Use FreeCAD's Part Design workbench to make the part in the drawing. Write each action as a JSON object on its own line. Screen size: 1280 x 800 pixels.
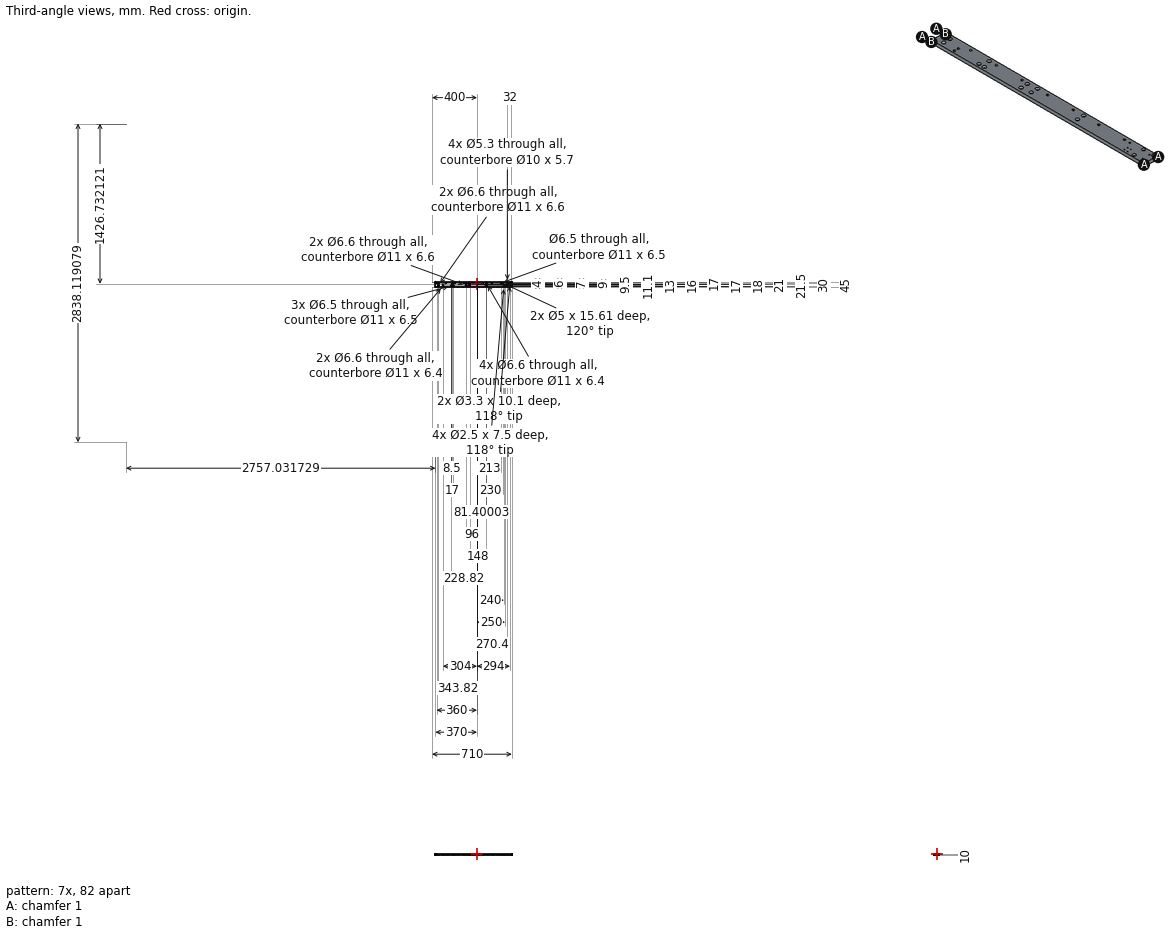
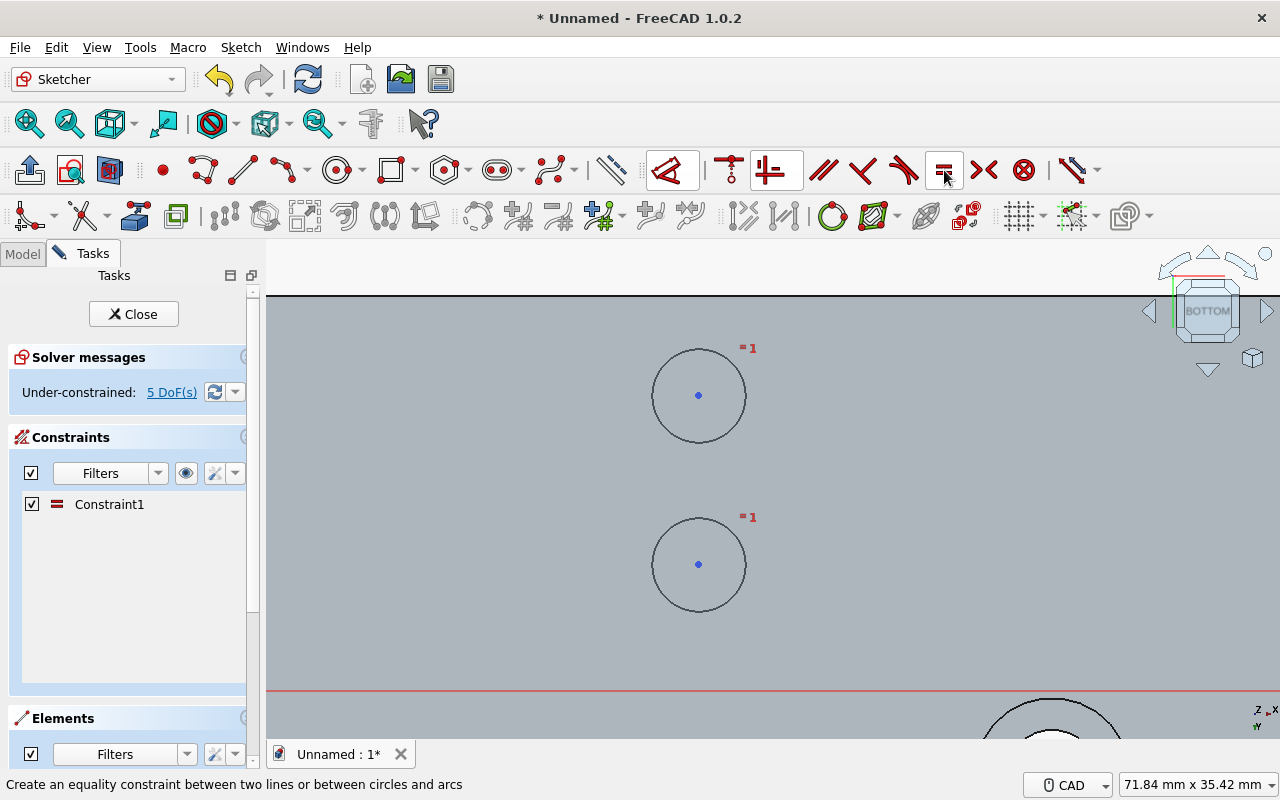
{"action": "left_click", "coordinate": [699, 396]}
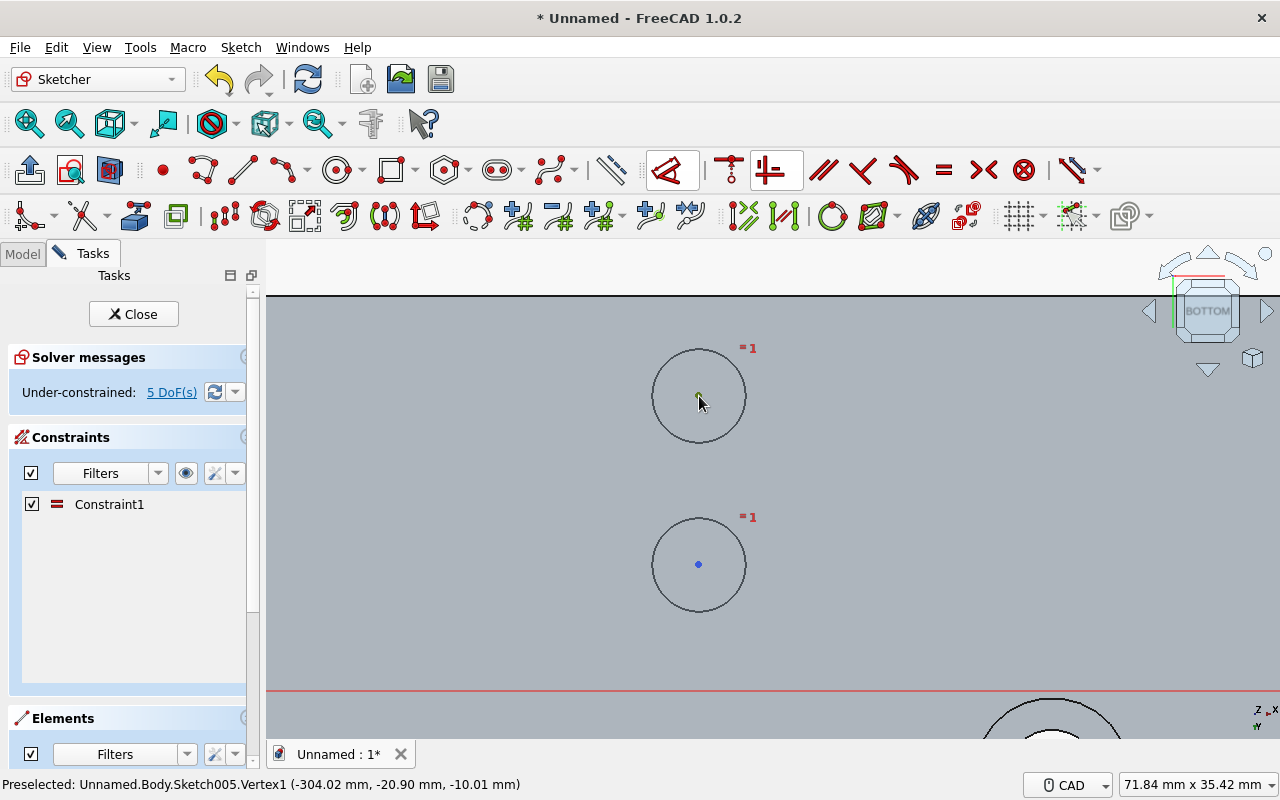
{"action": "left_click", "coordinate": [699, 565]}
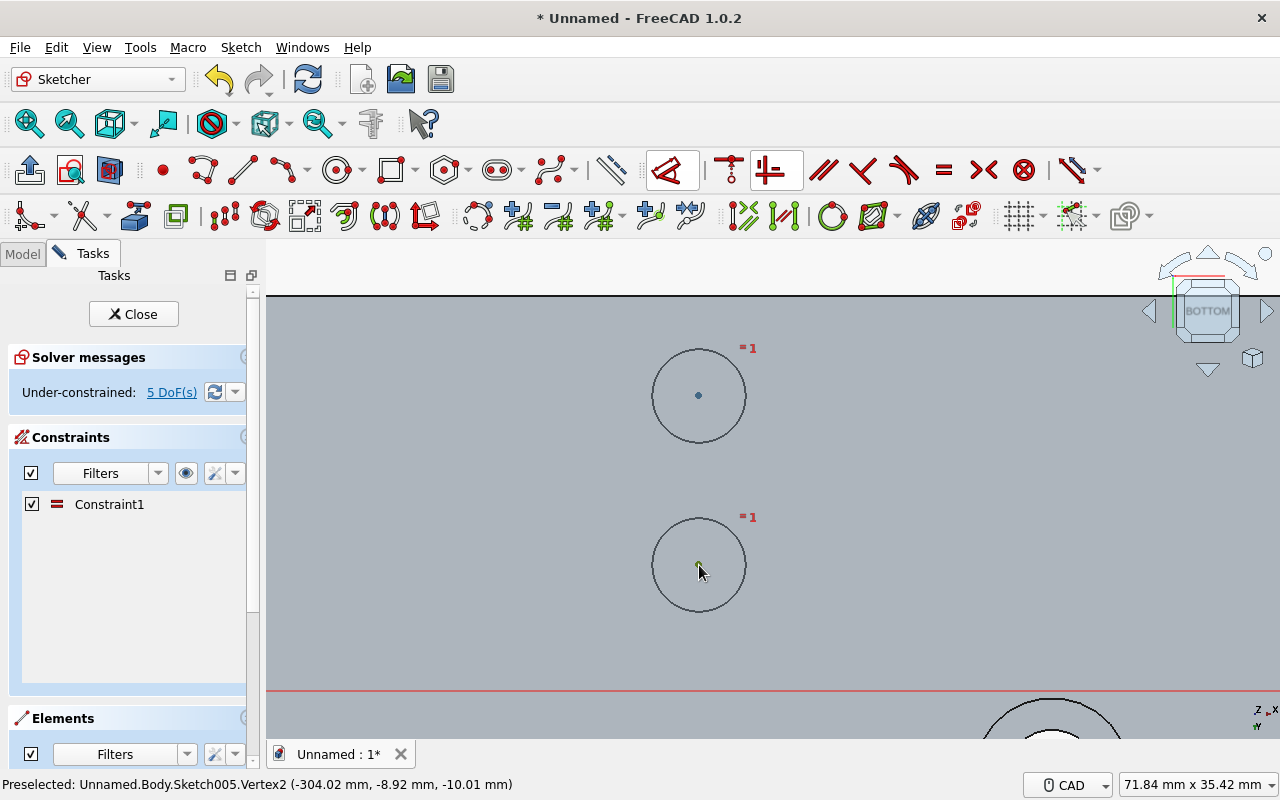
{"action": "left_click", "coordinate": [798, 170]}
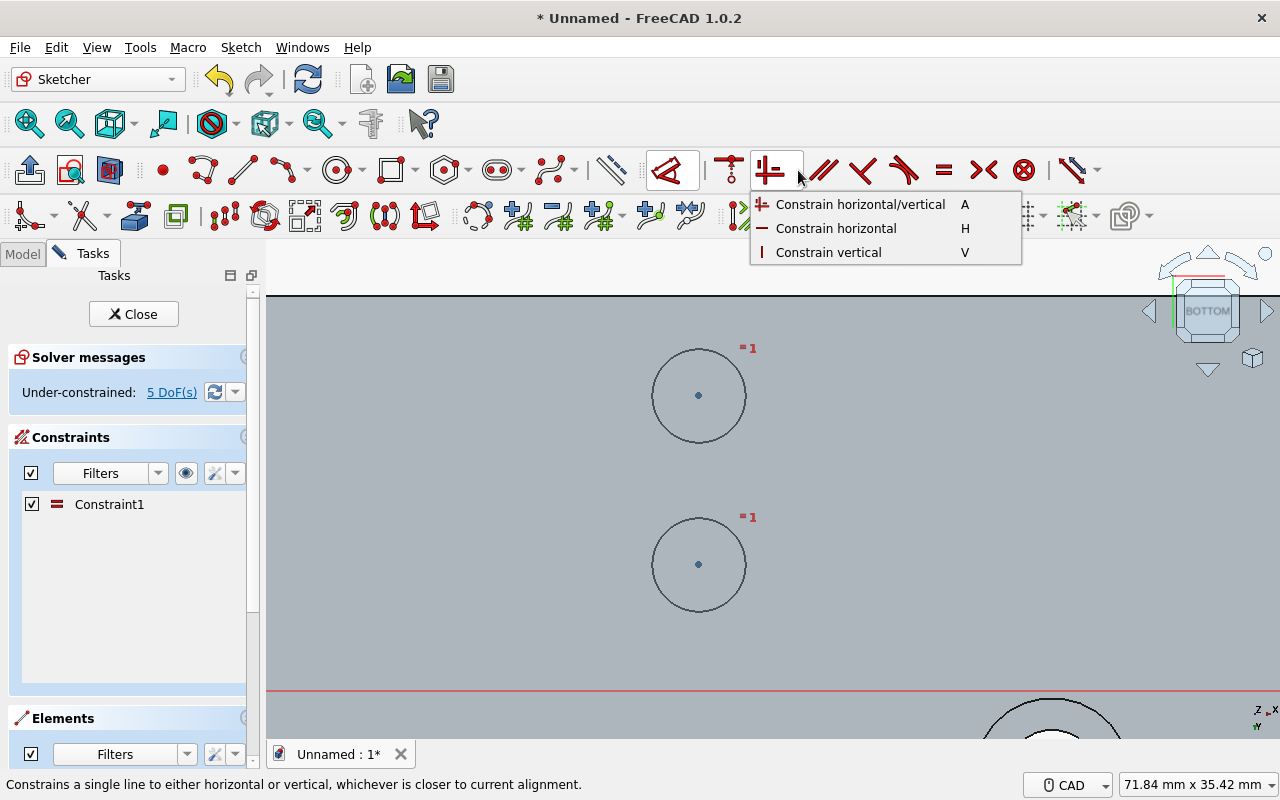
{"action": "left_click", "coordinate": [886, 252]}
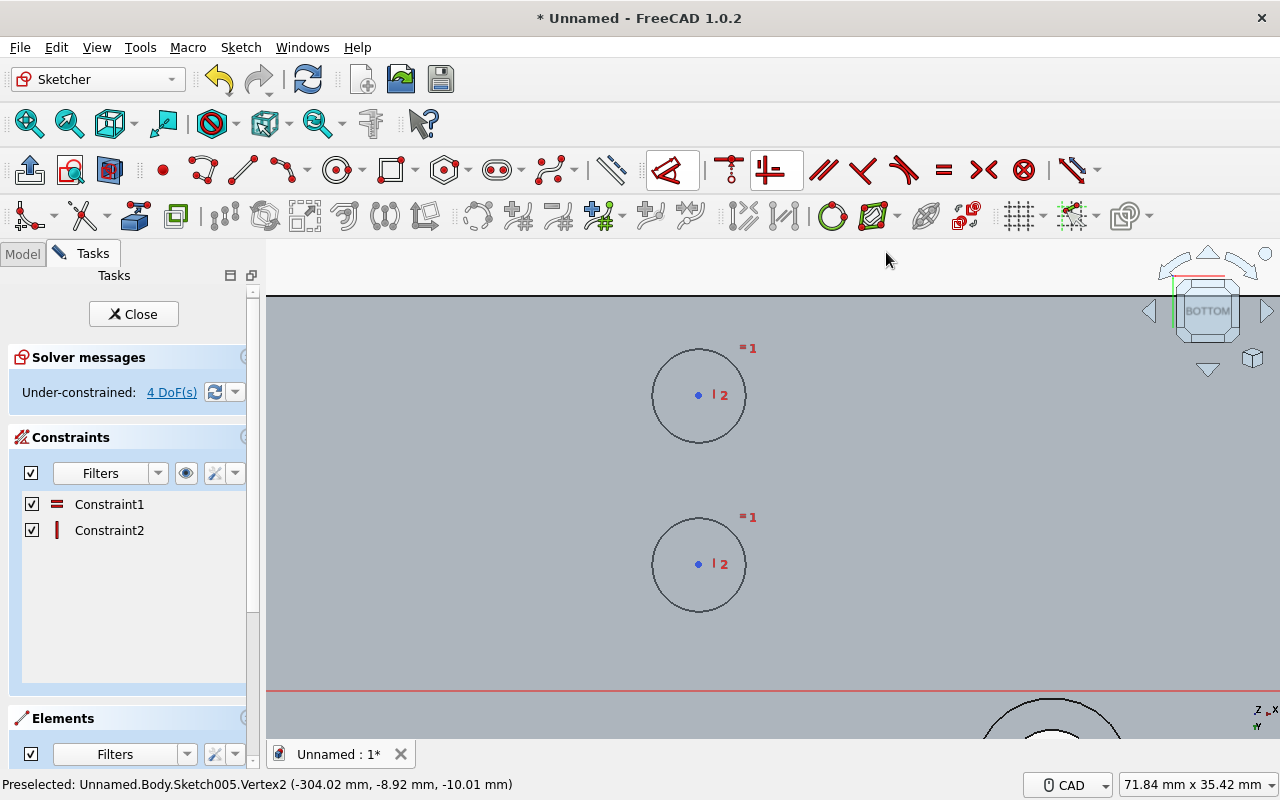
{"action": "left_click", "coordinate": [732, 363]}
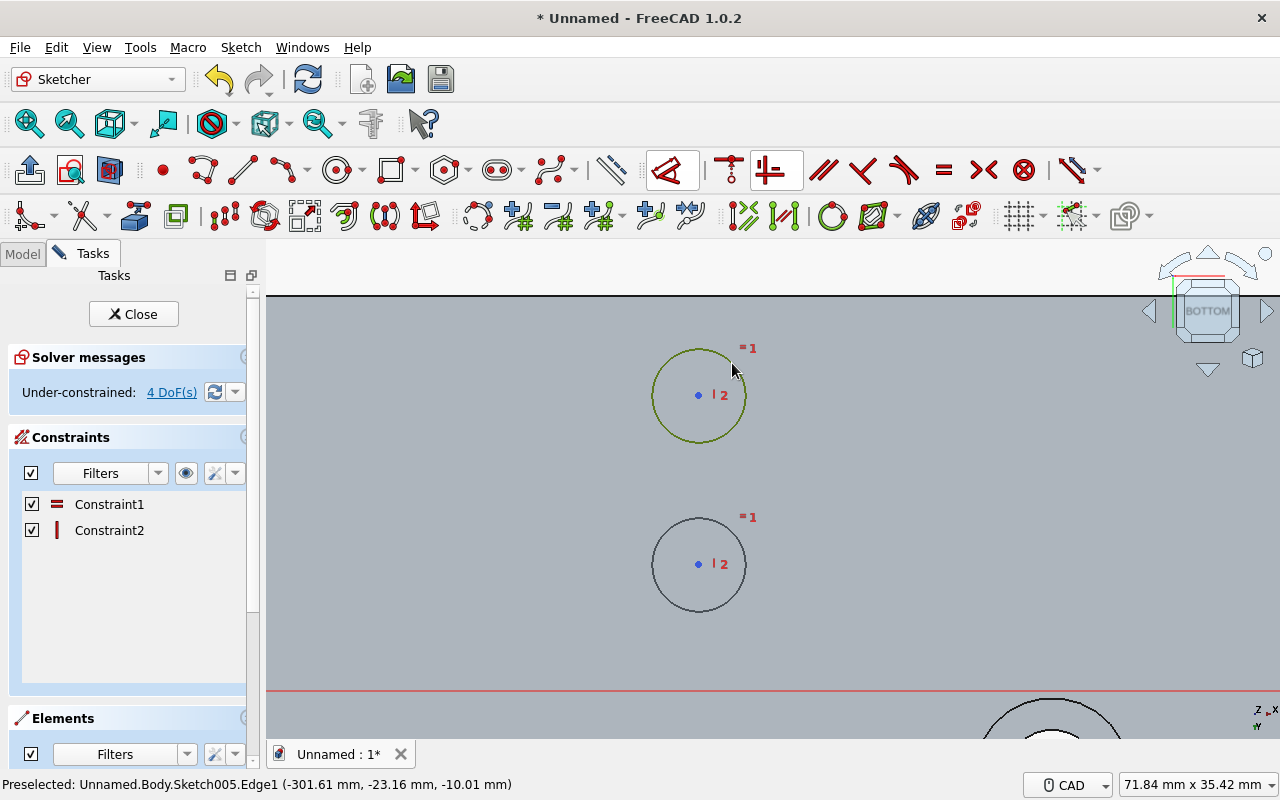
{"action": "left_click", "coordinate": [694, 170]}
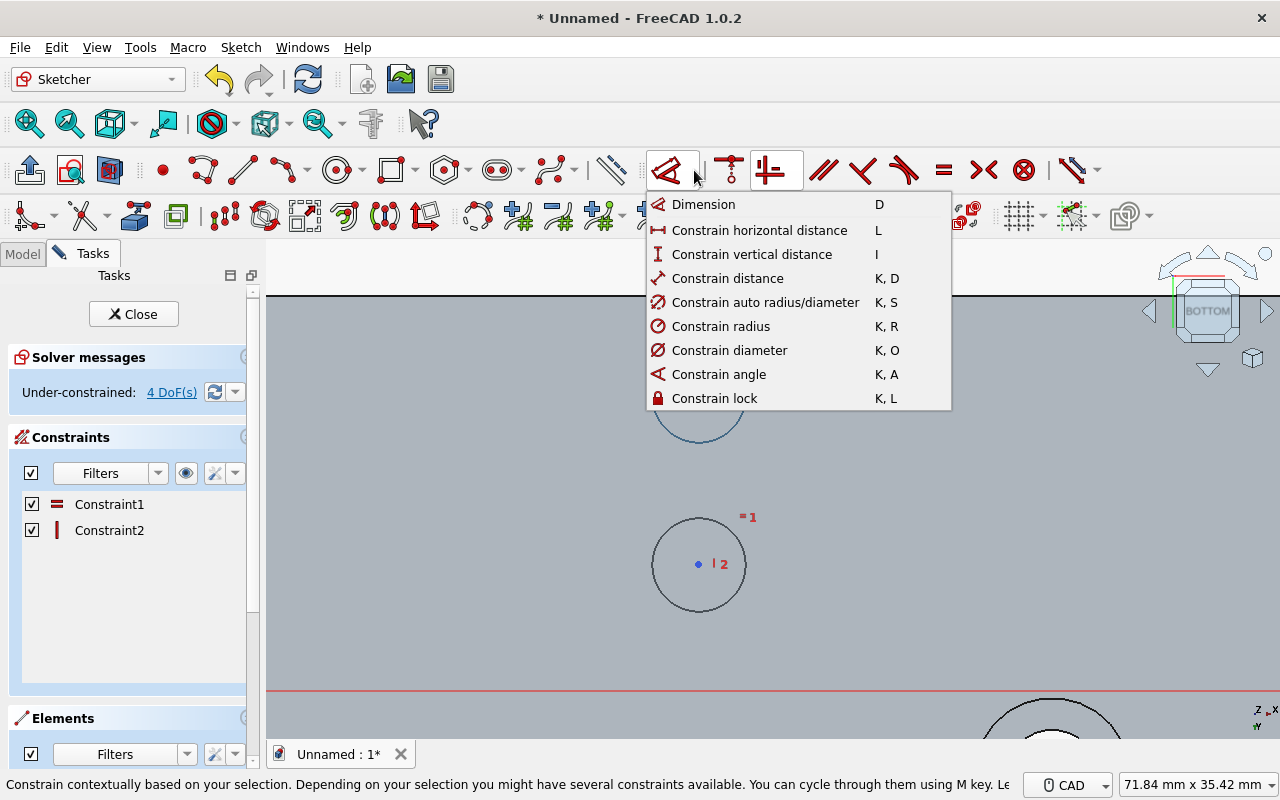
{"action": "left_click", "coordinate": [799, 350]}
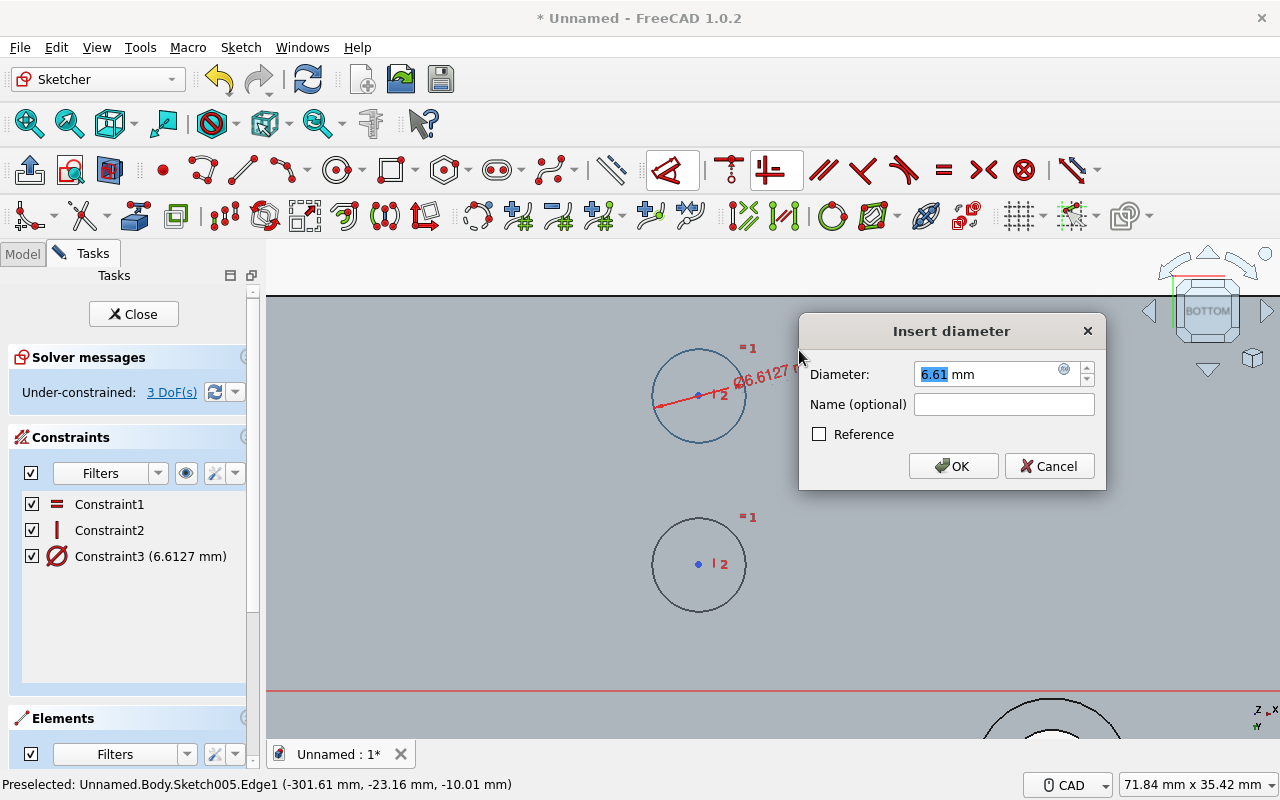
{"action": "type", "text": "6.6"}
{"action": "key", "text": "Return"}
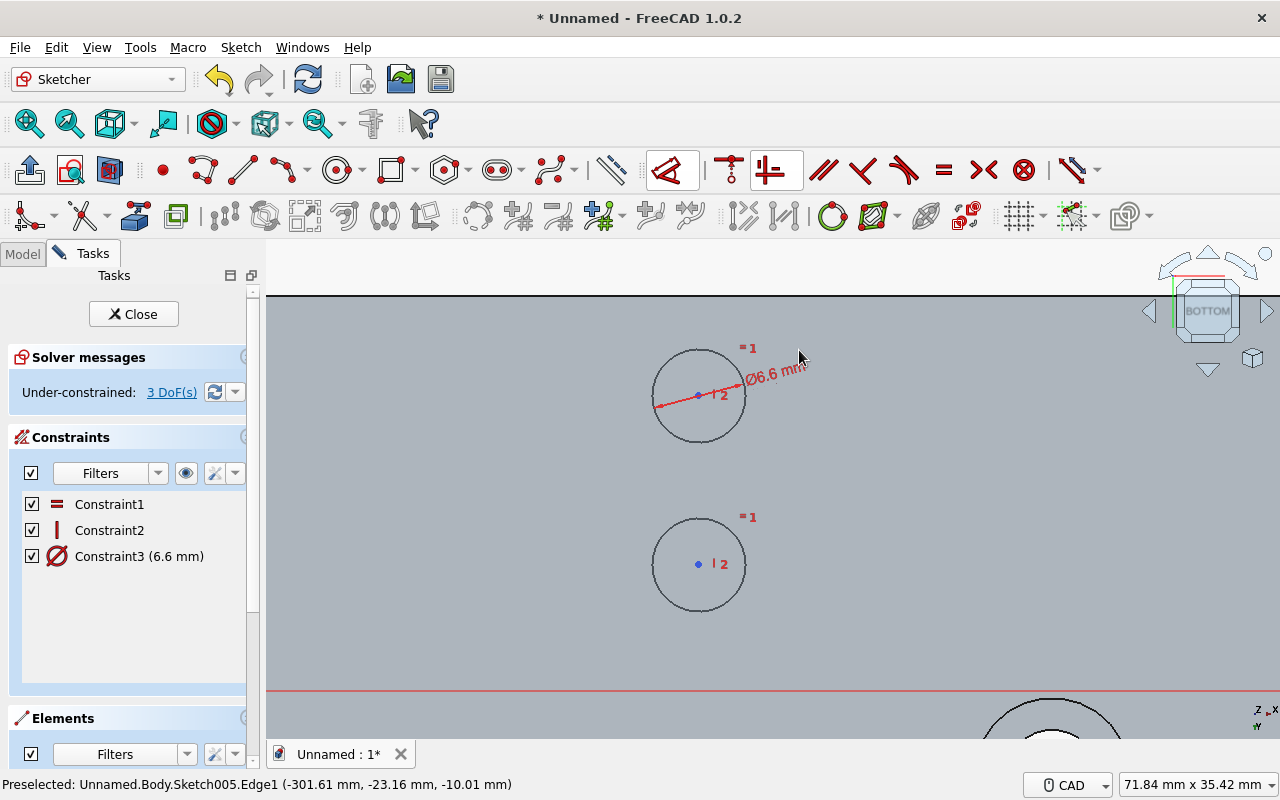
{"action": "left_click", "coordinate": [699, 565]}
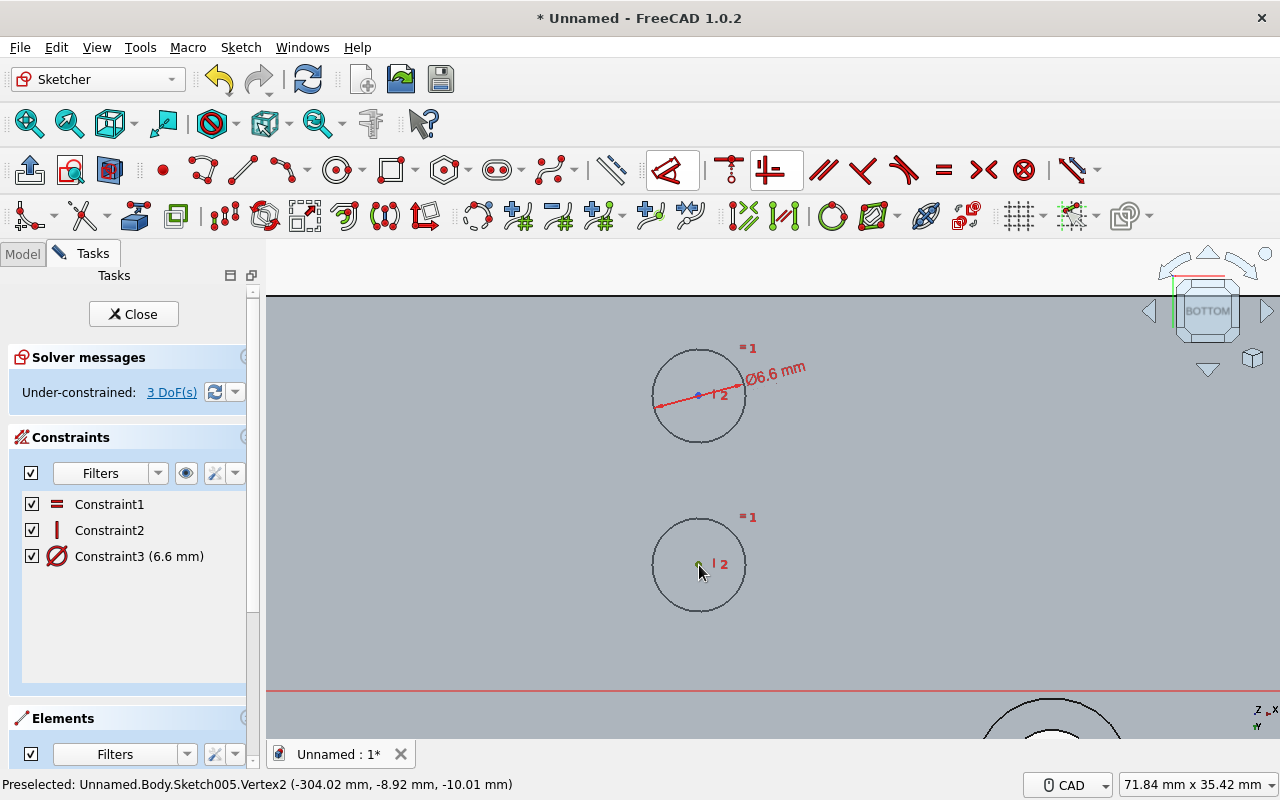
{"action": "left_click", "coordinate": [694, 170]}